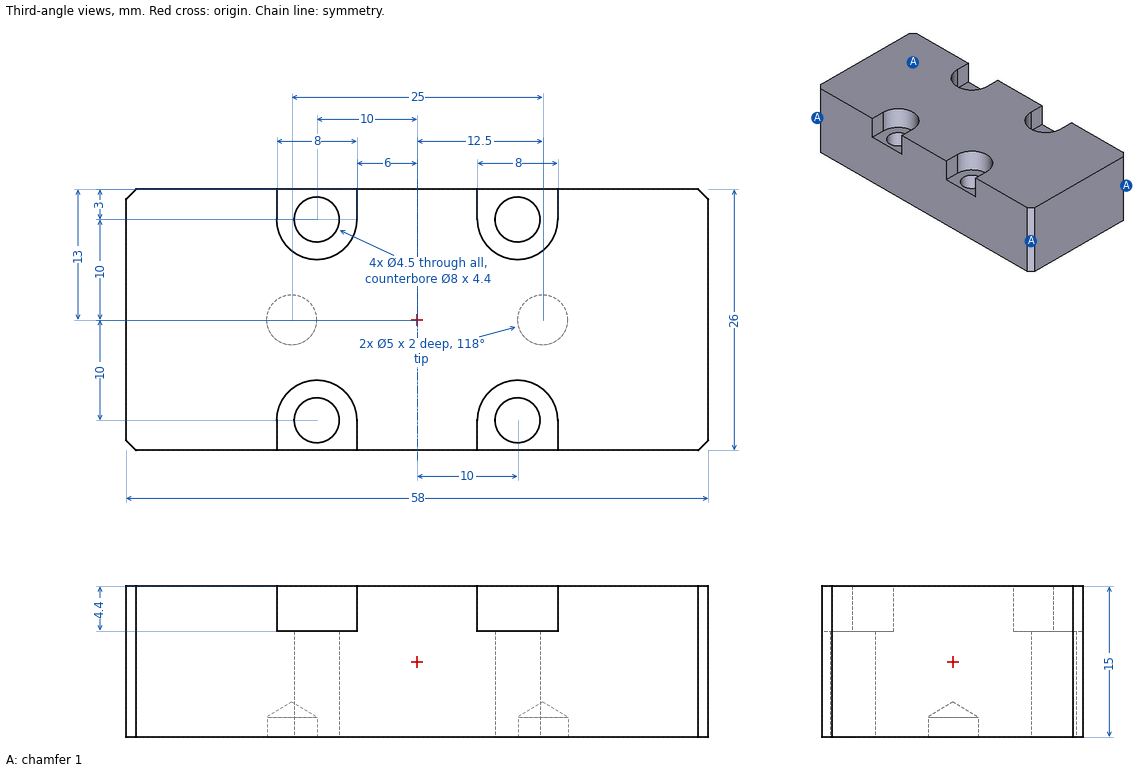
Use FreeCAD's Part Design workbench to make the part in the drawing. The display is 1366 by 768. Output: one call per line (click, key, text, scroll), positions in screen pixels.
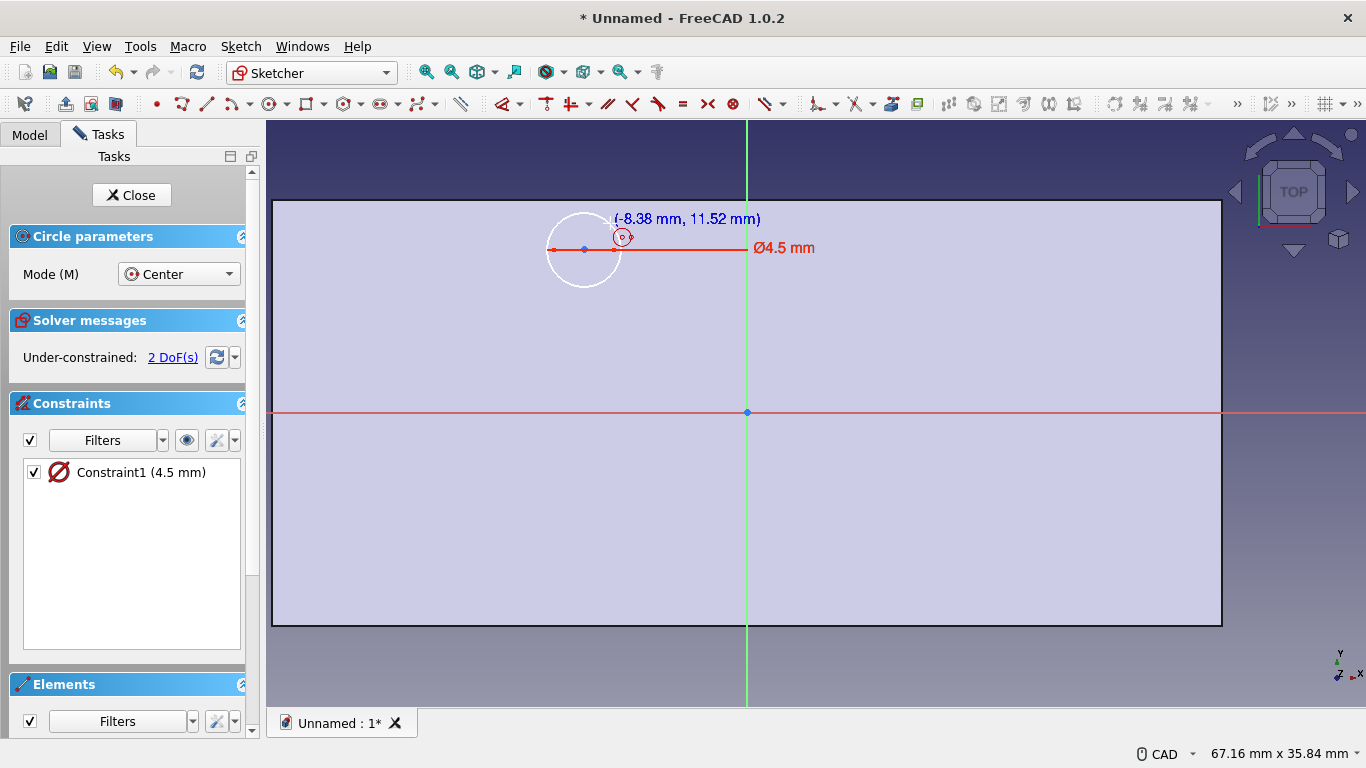
click(584, 576)
move(610, 550)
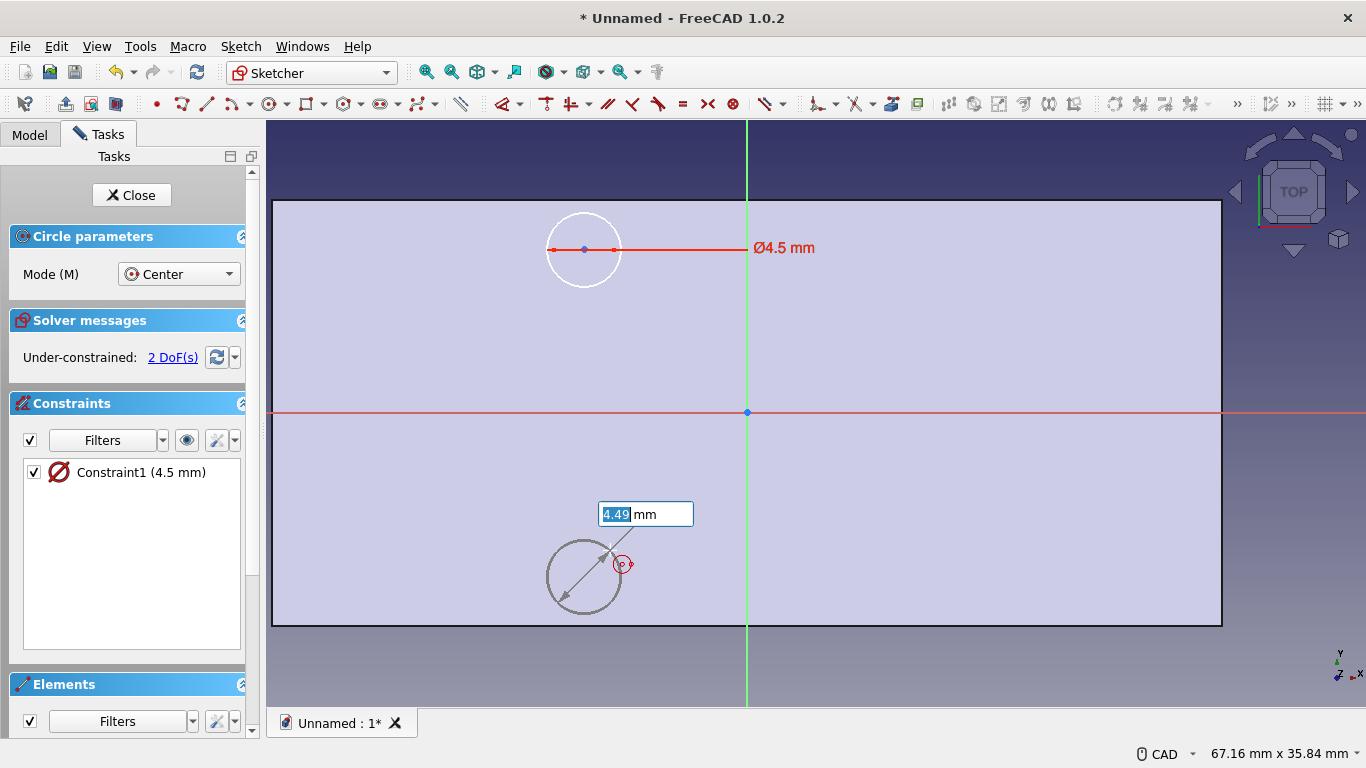
text(4.5)
key(Return)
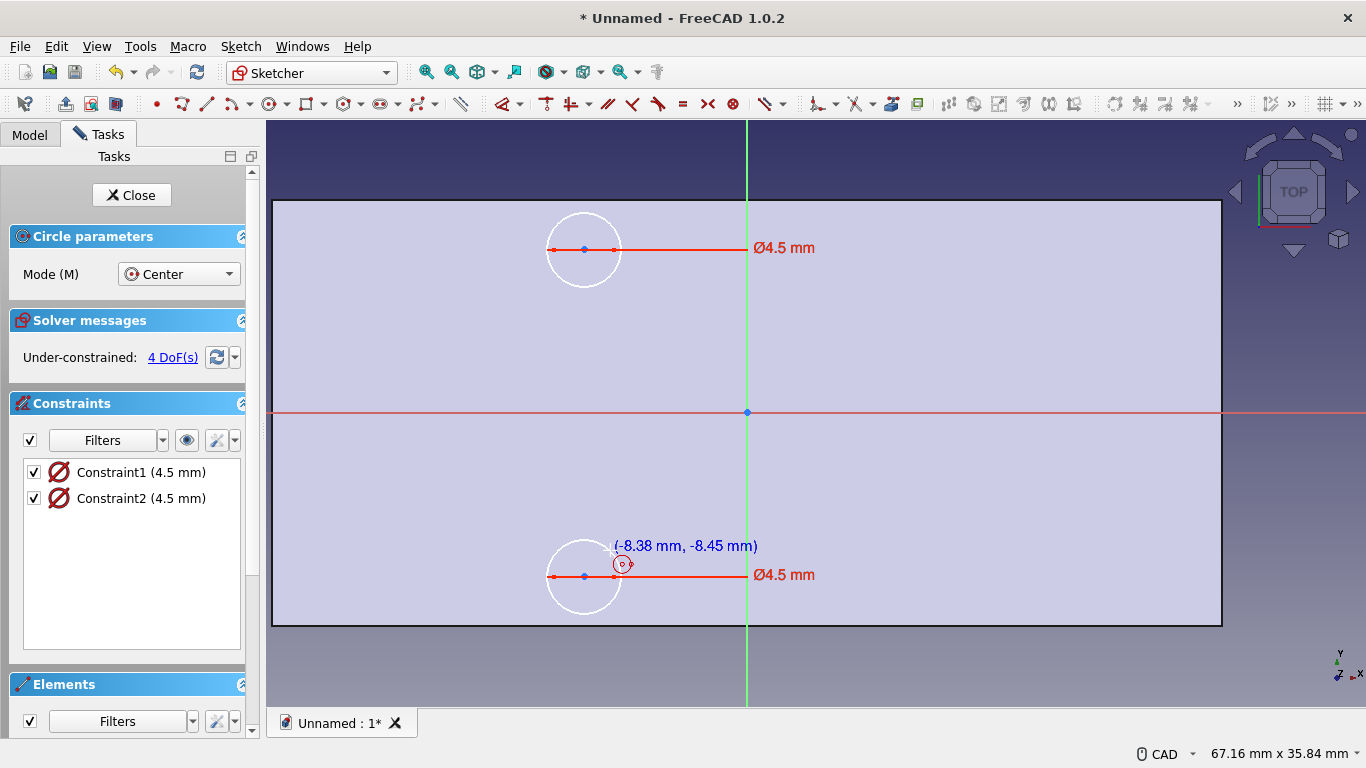
click(911, 576)
move(937, 550)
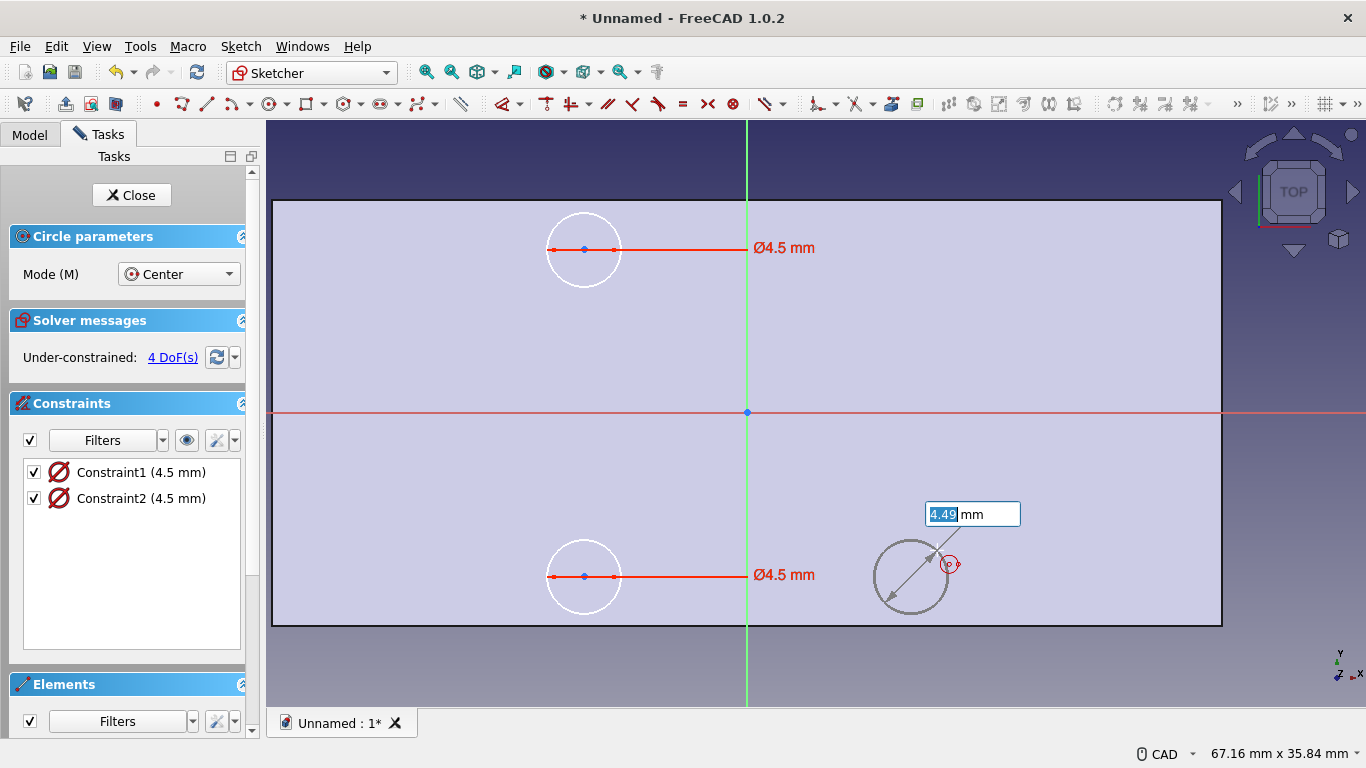
text(4.5)
key(Return)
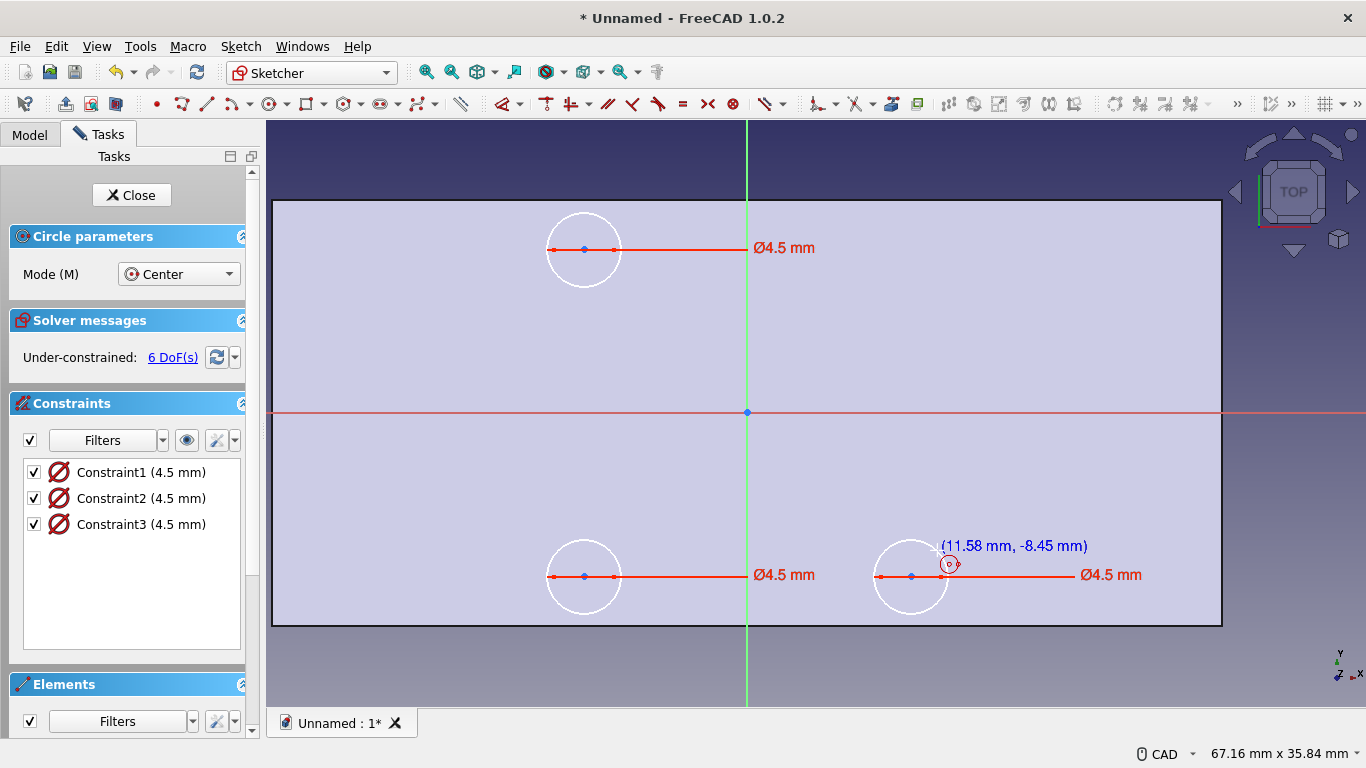
click(911, 249)
move(937, 223)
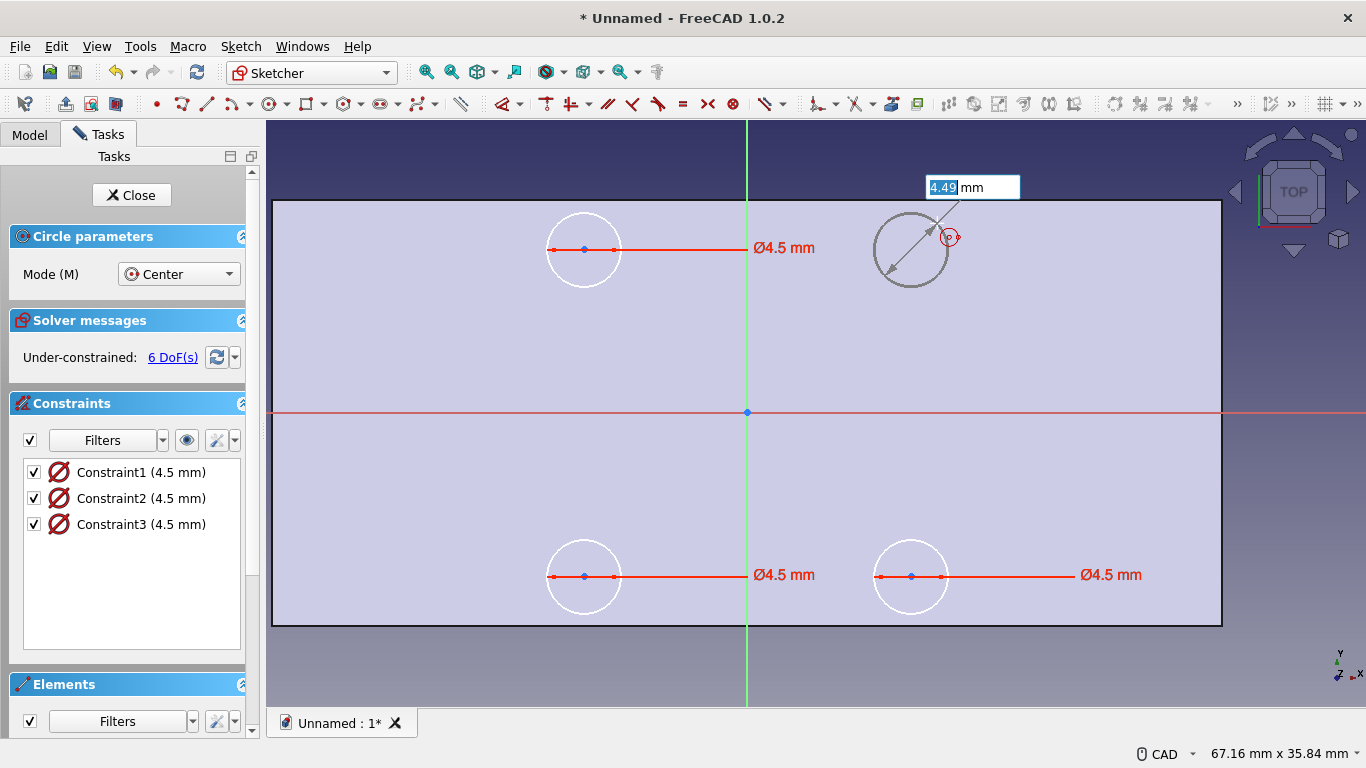
text(4.5)
key(Return)
key(Escape)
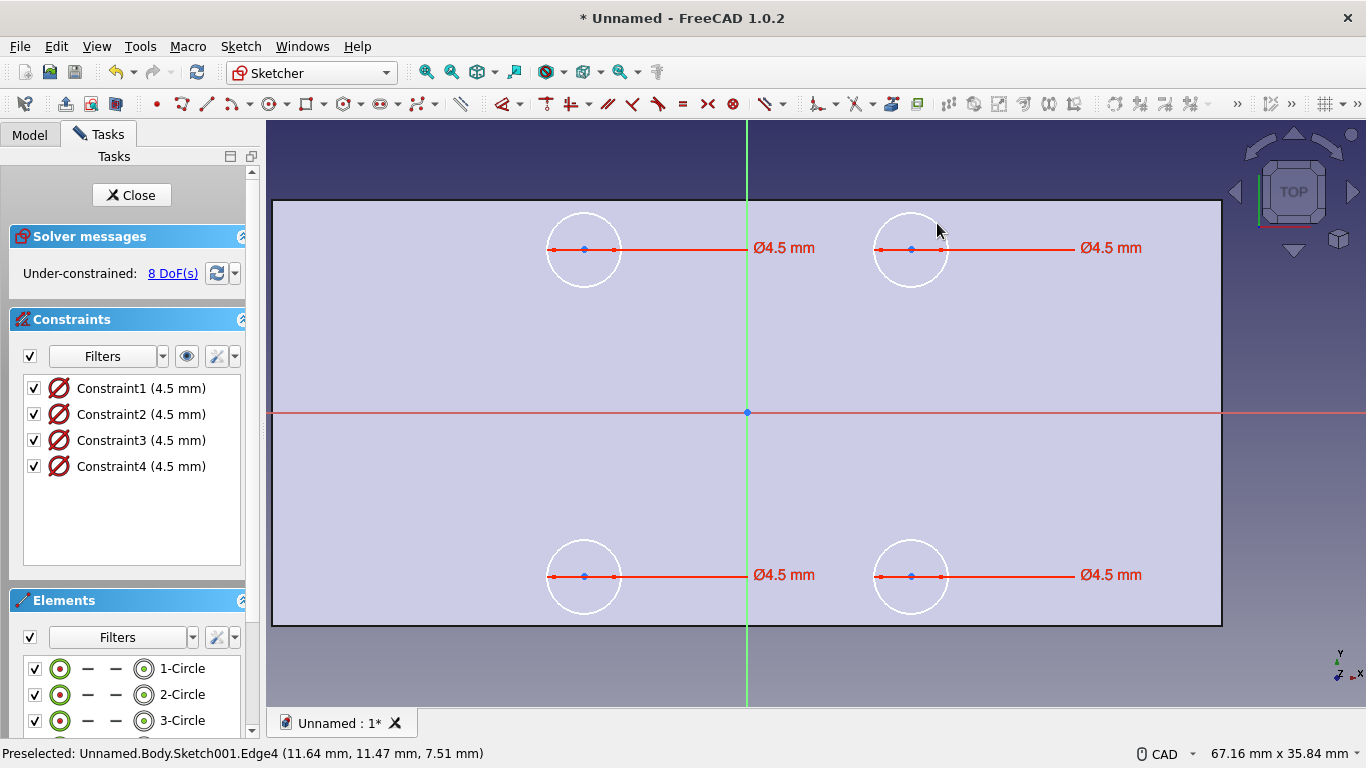
click(584, 250)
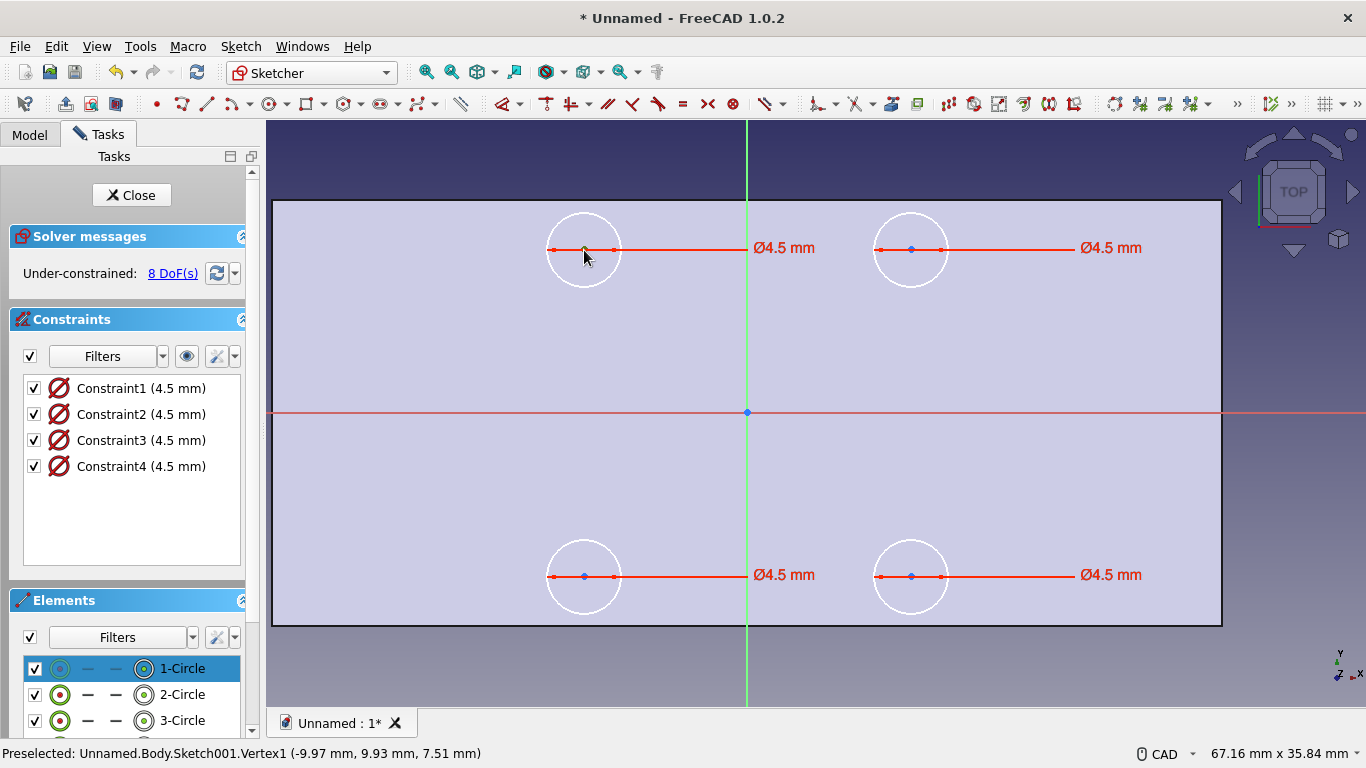
click(584, 577)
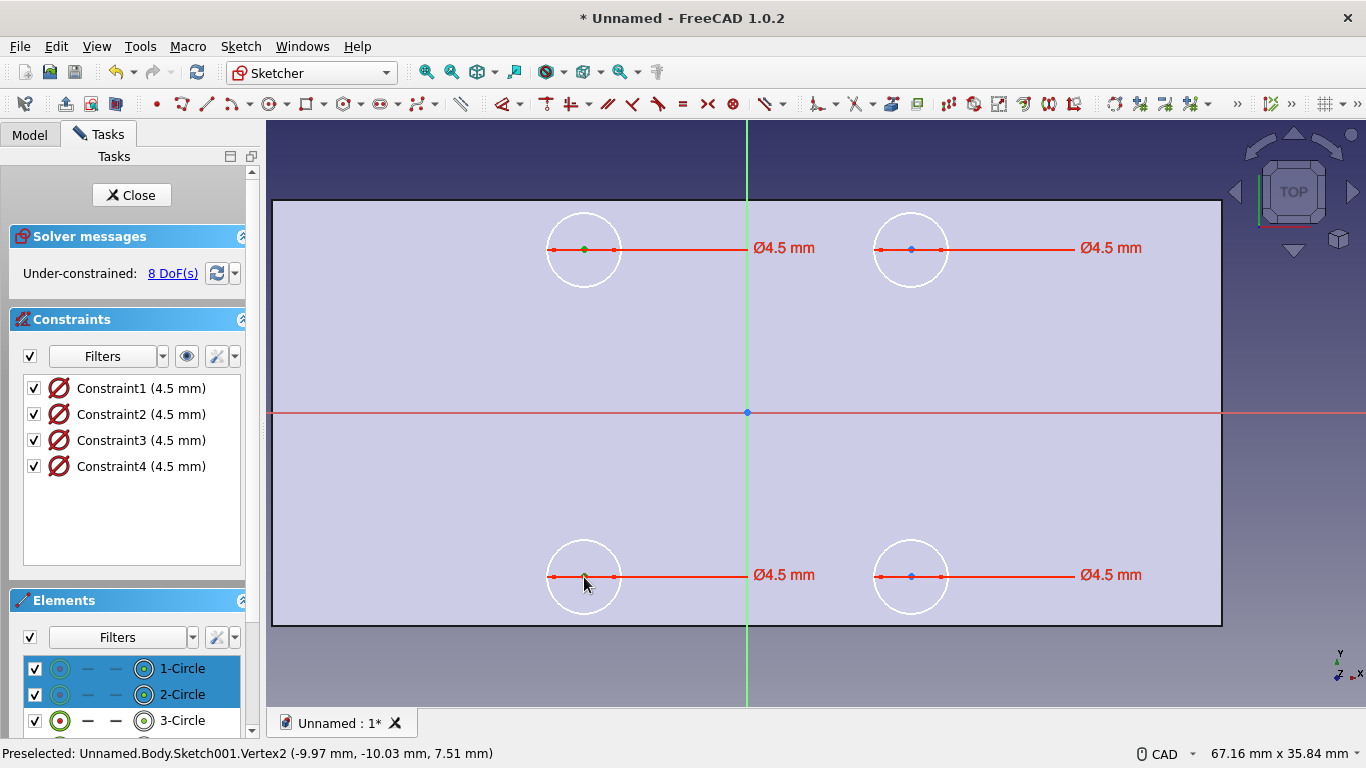
key(v)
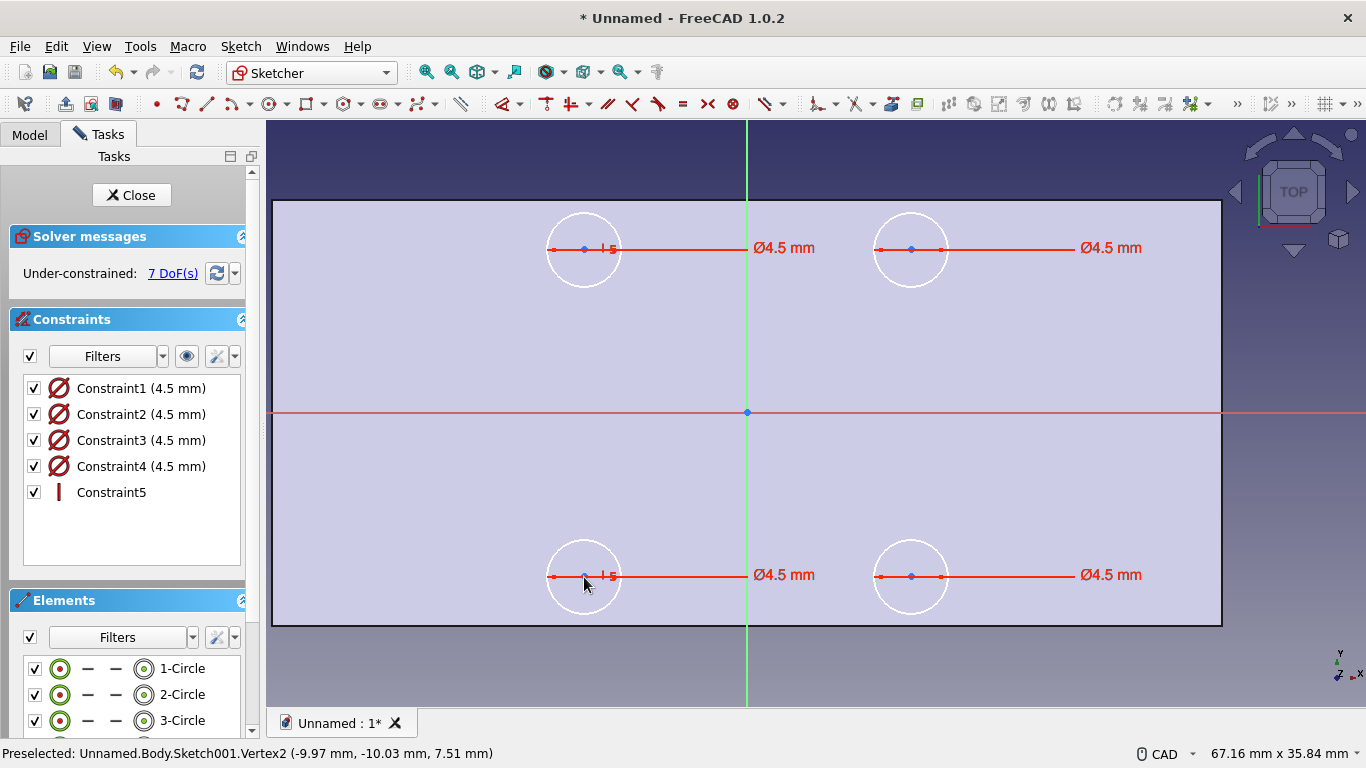
click(584, 577)